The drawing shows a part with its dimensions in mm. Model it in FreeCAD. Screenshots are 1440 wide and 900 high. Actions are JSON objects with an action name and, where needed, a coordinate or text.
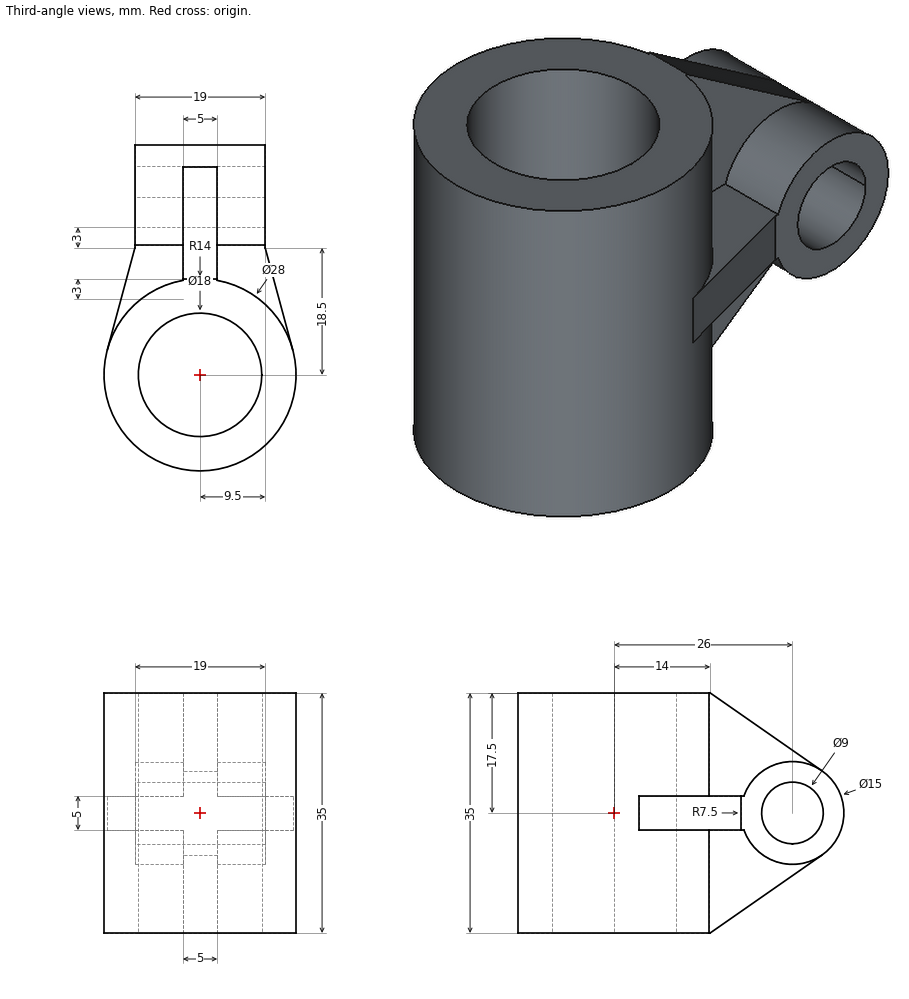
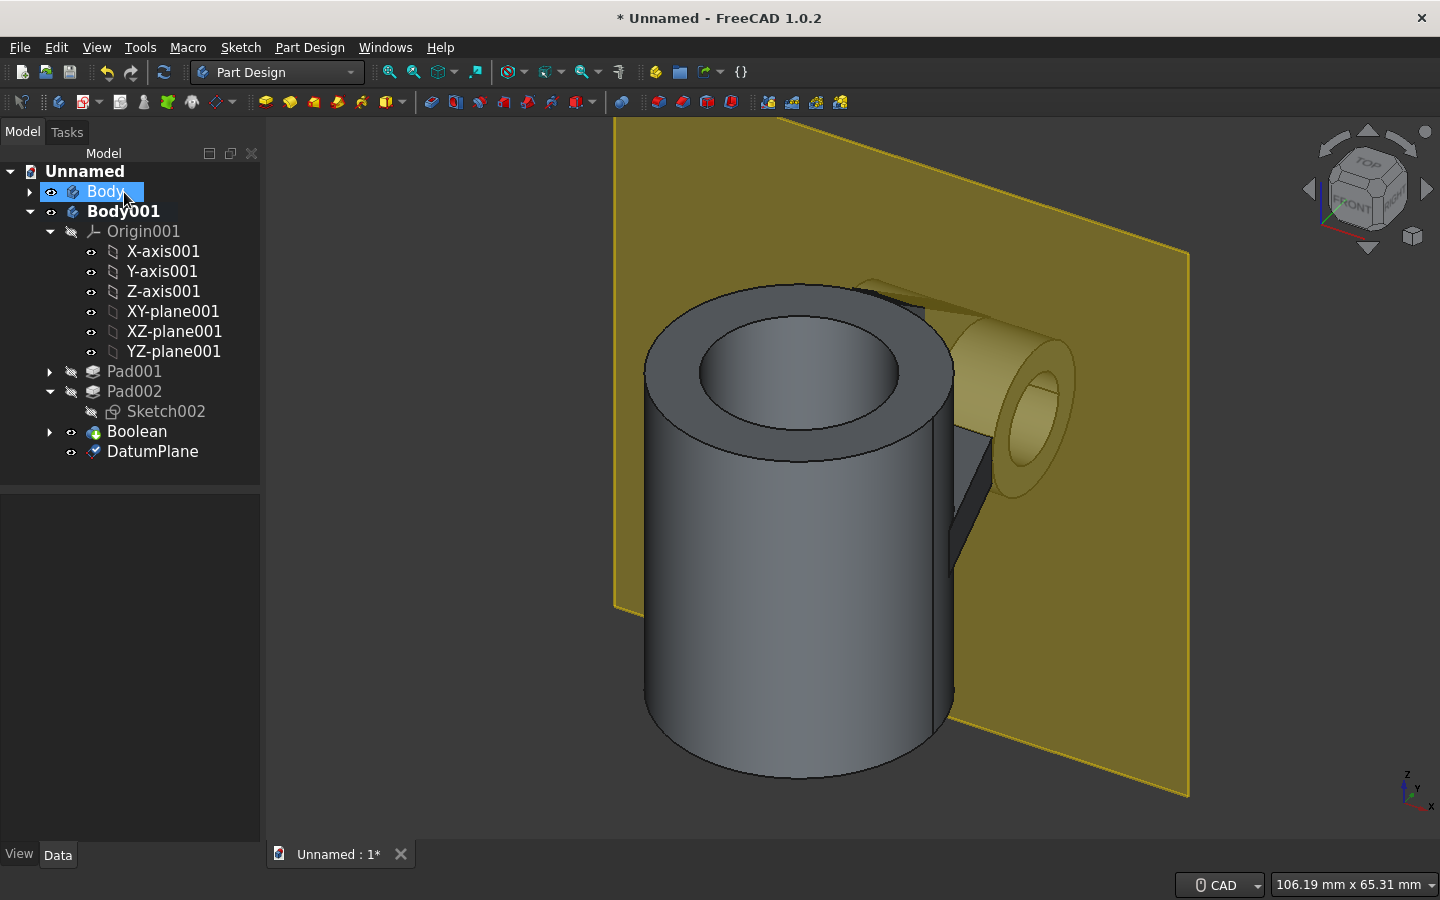
{"action": "left_click", "coordinate": [116, 452]}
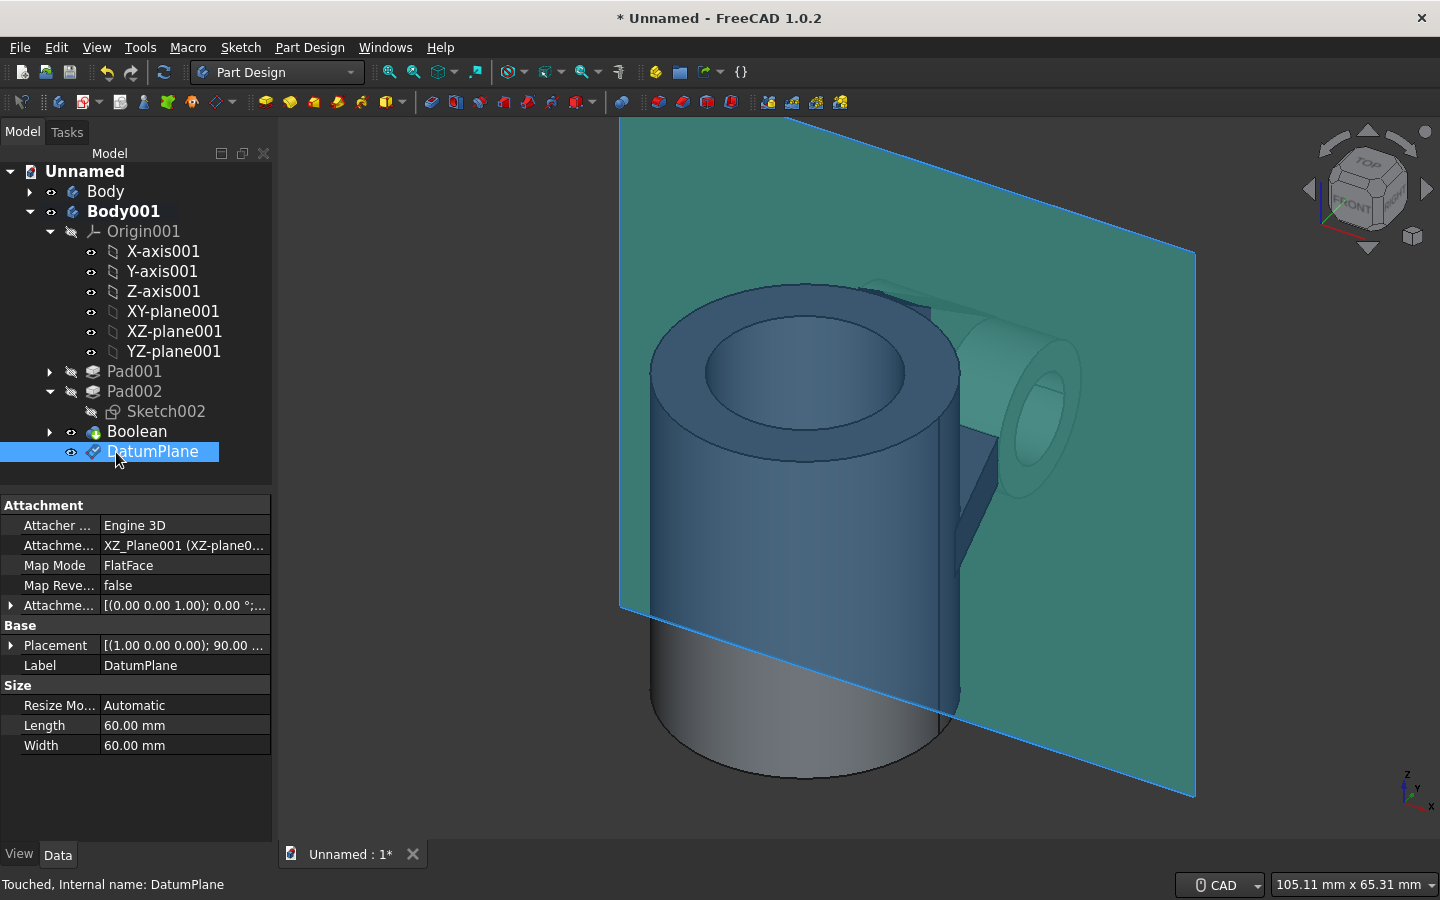
{"action": "left_click", "coordinate": [84, 102]}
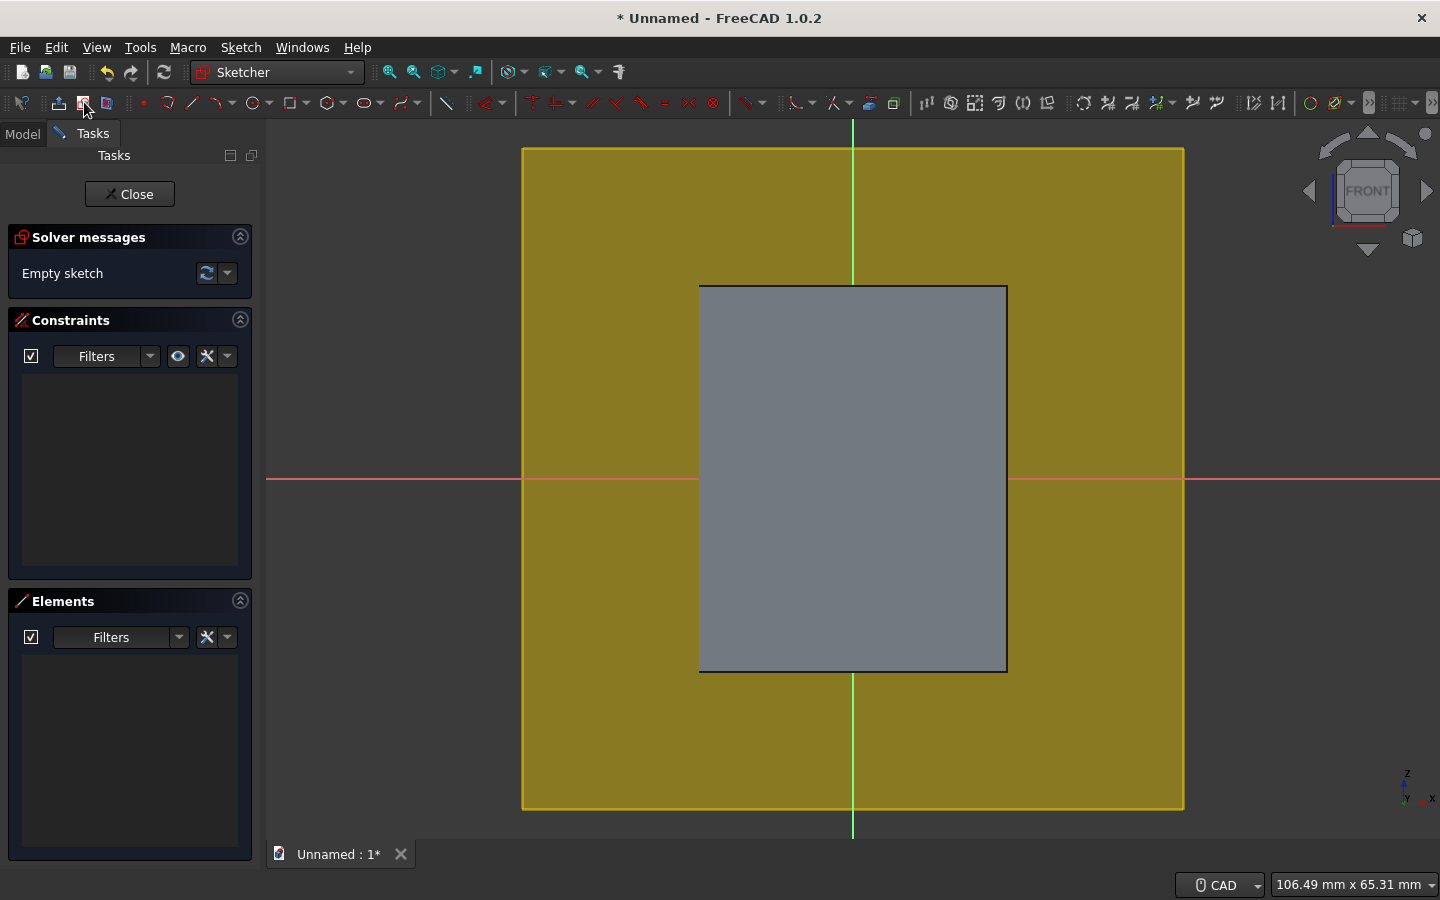
{"action": "key", "text": "q s"}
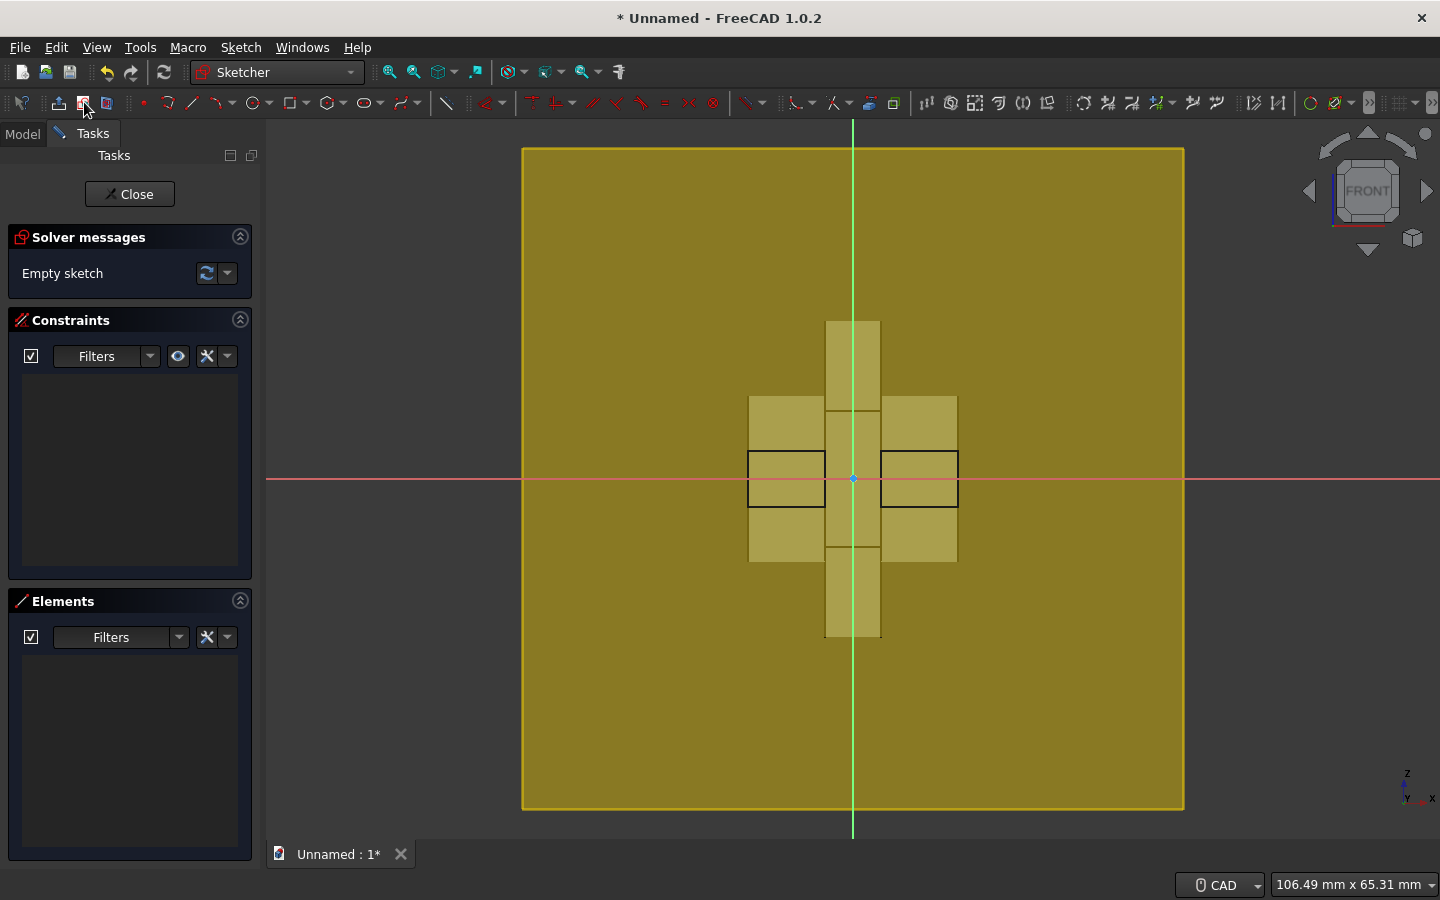
{"action": "scroll", "coordinate": [883, 479], "scroll_direction": "up", "scroll_amount": 6}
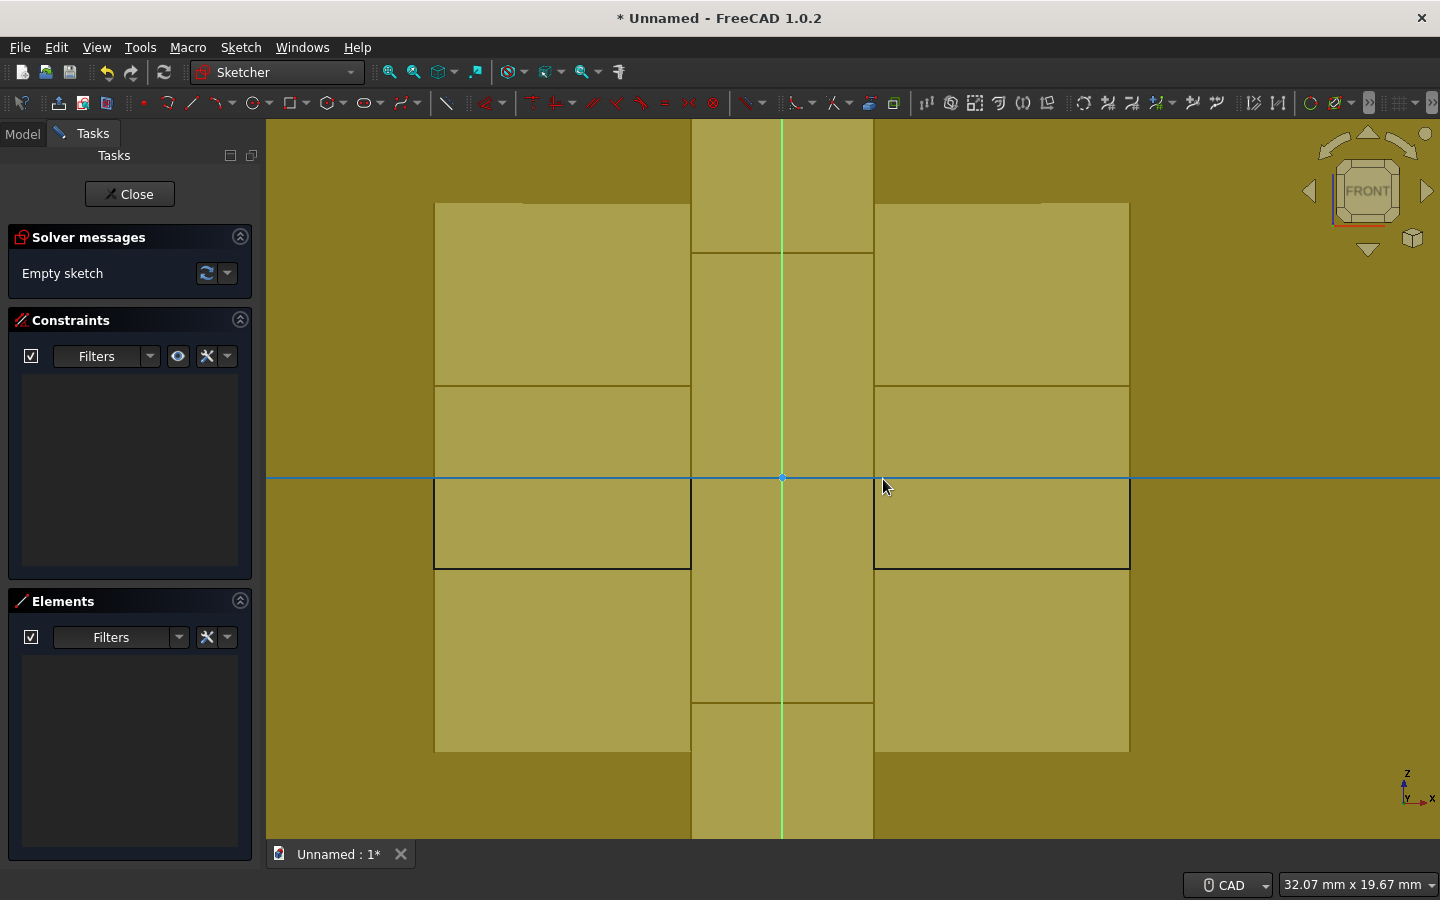
{"action": "key", "text": "g v"}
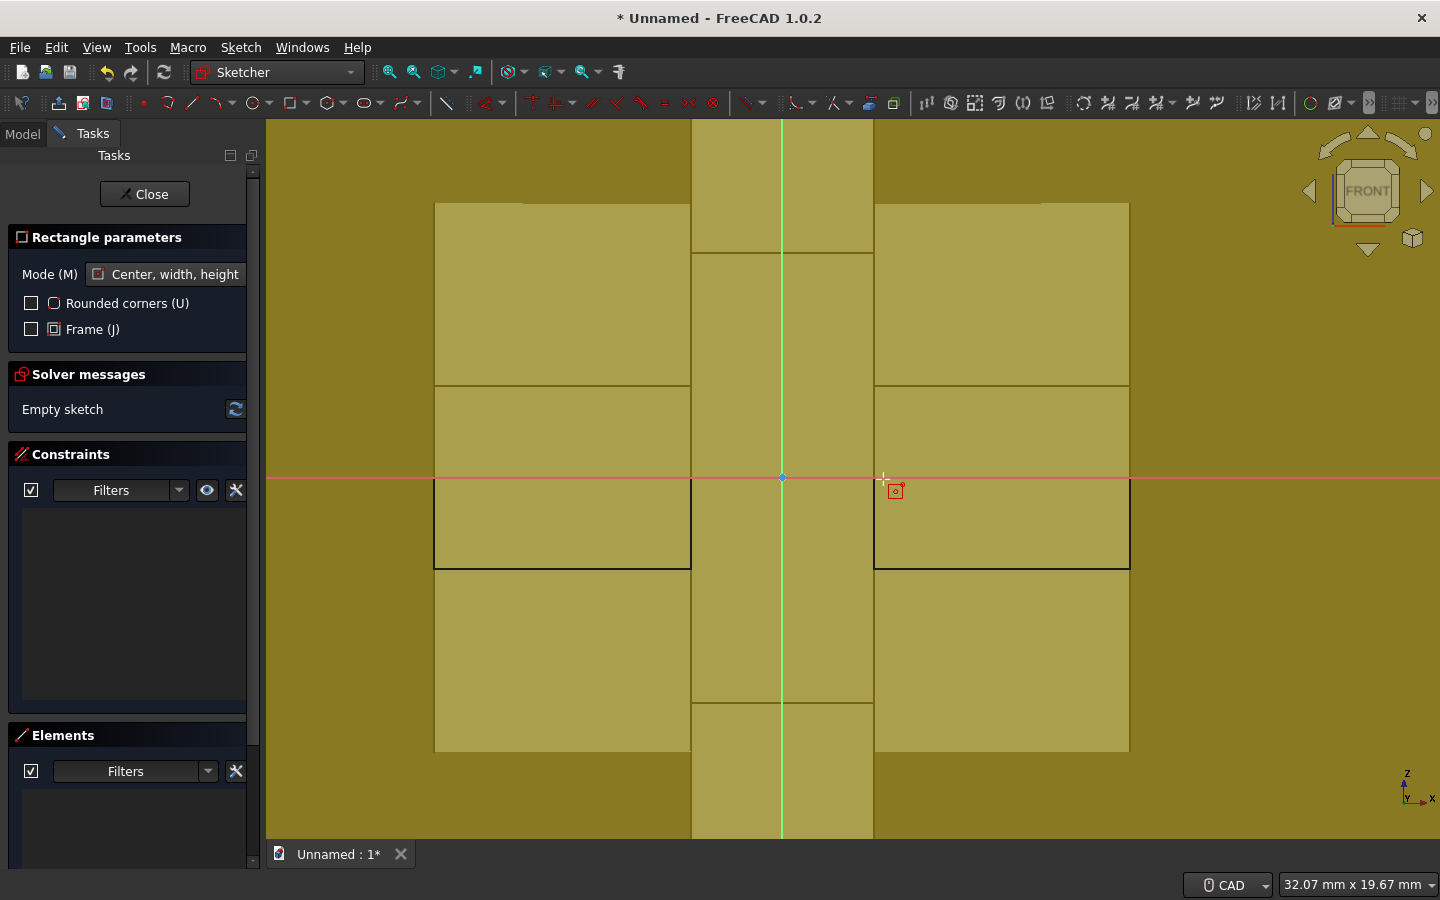
{"action": "left_click", "coordinate": [782, 478]}
{"action": "left_click", "coordinate": [1130, 386]}
{"action": "key", "text": "Escape"}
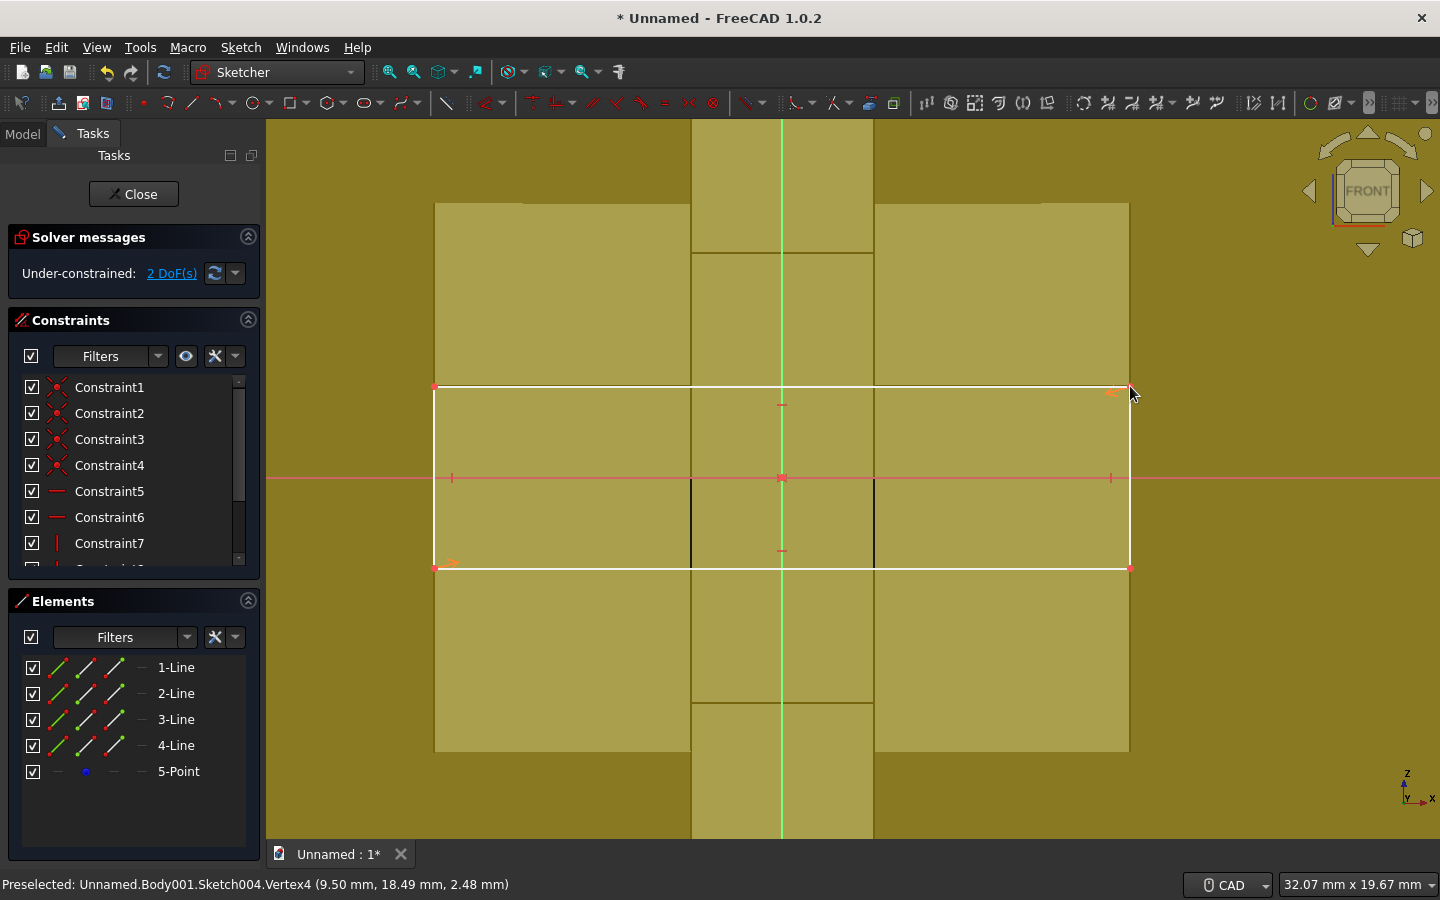
{"action": "key", "text": "d"}